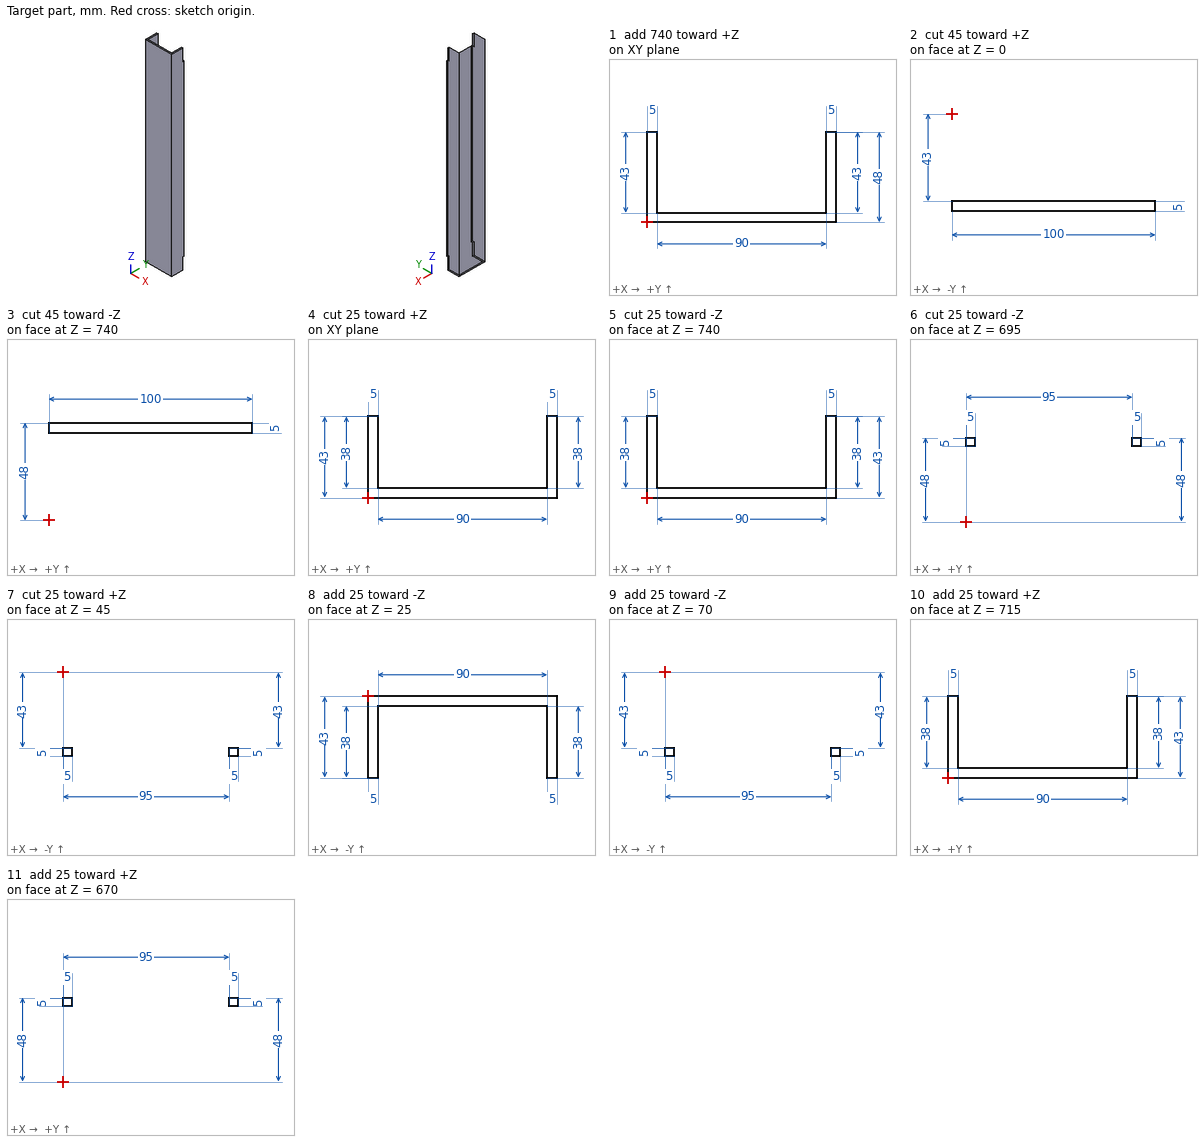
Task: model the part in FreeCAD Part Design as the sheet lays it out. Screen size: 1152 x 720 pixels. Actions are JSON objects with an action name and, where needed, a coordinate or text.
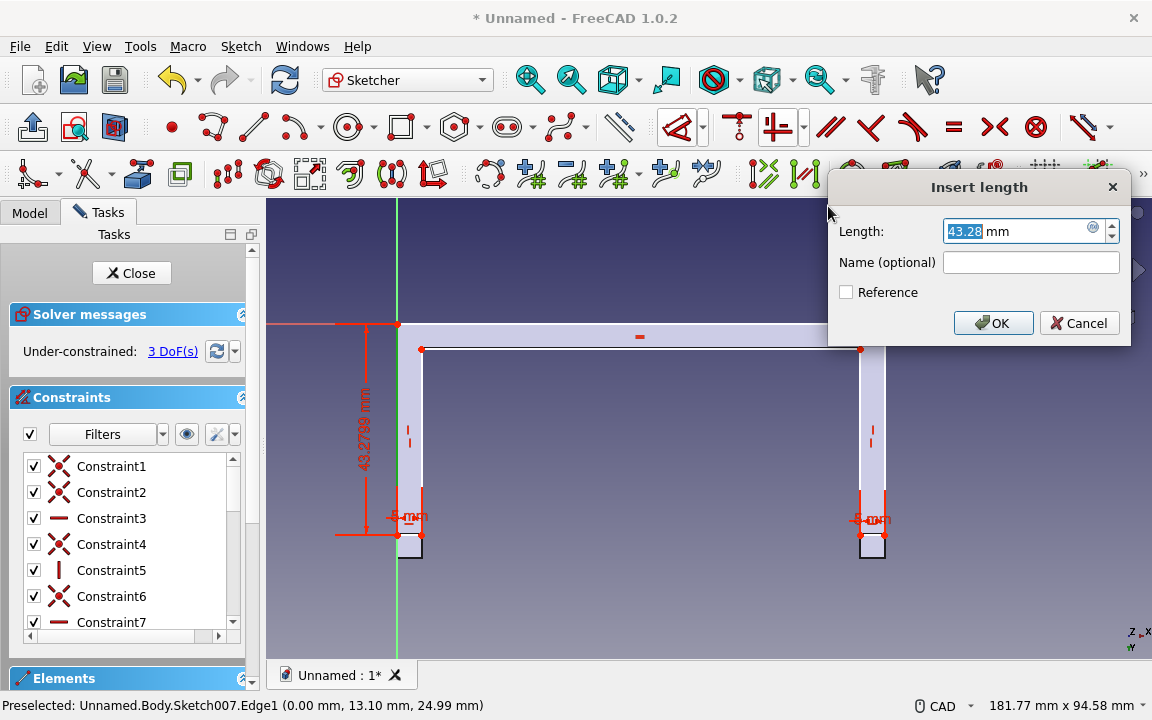
{"action": "type", "text": "43"}
{"action": "key", "text": "Return"}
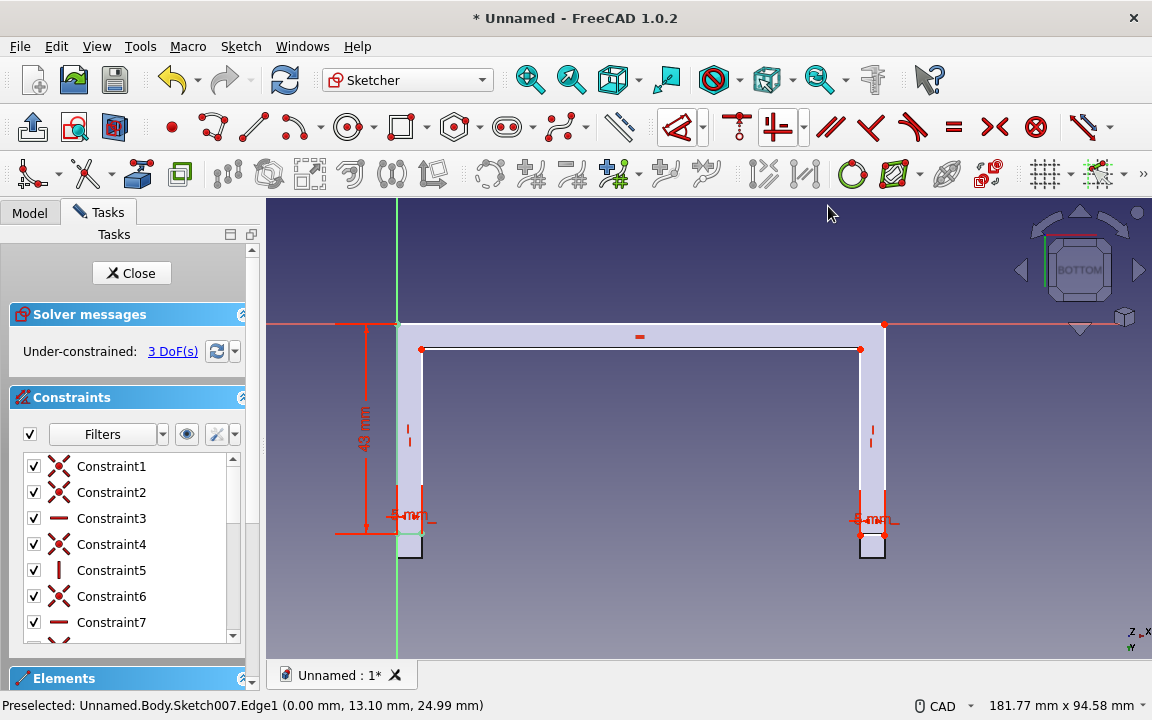
{"action": "left_click", "coordinate": [422, 478]}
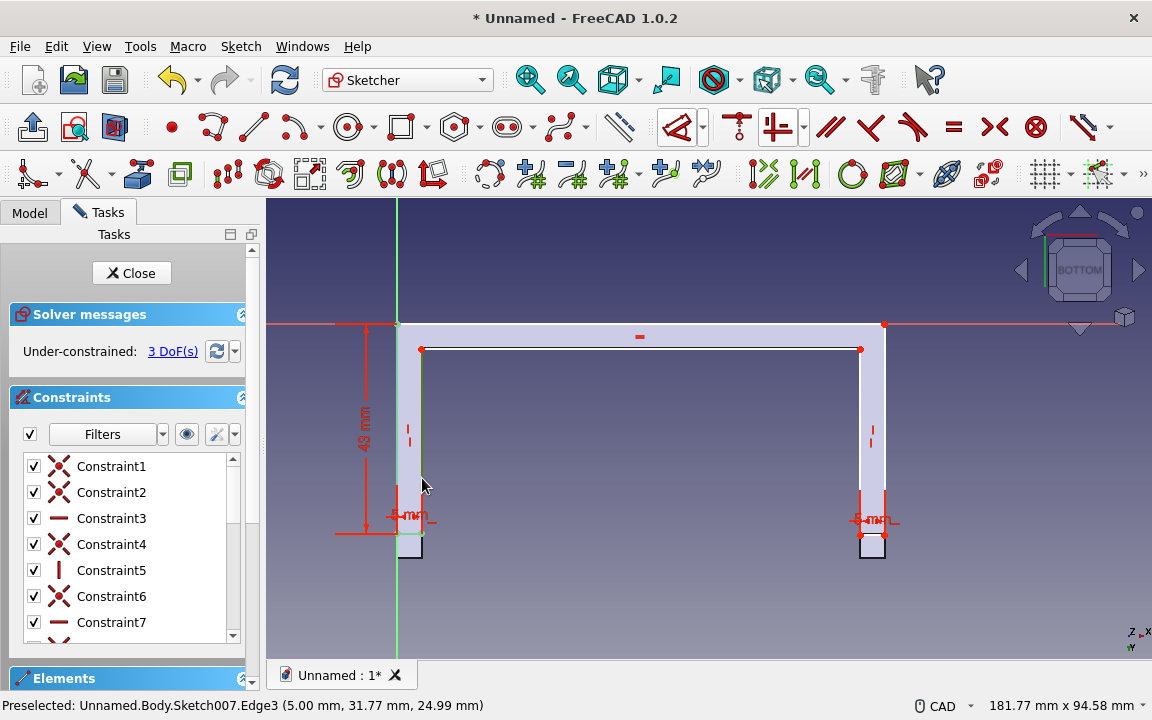
{"action": "left_click", "coordinate": [702, 128]}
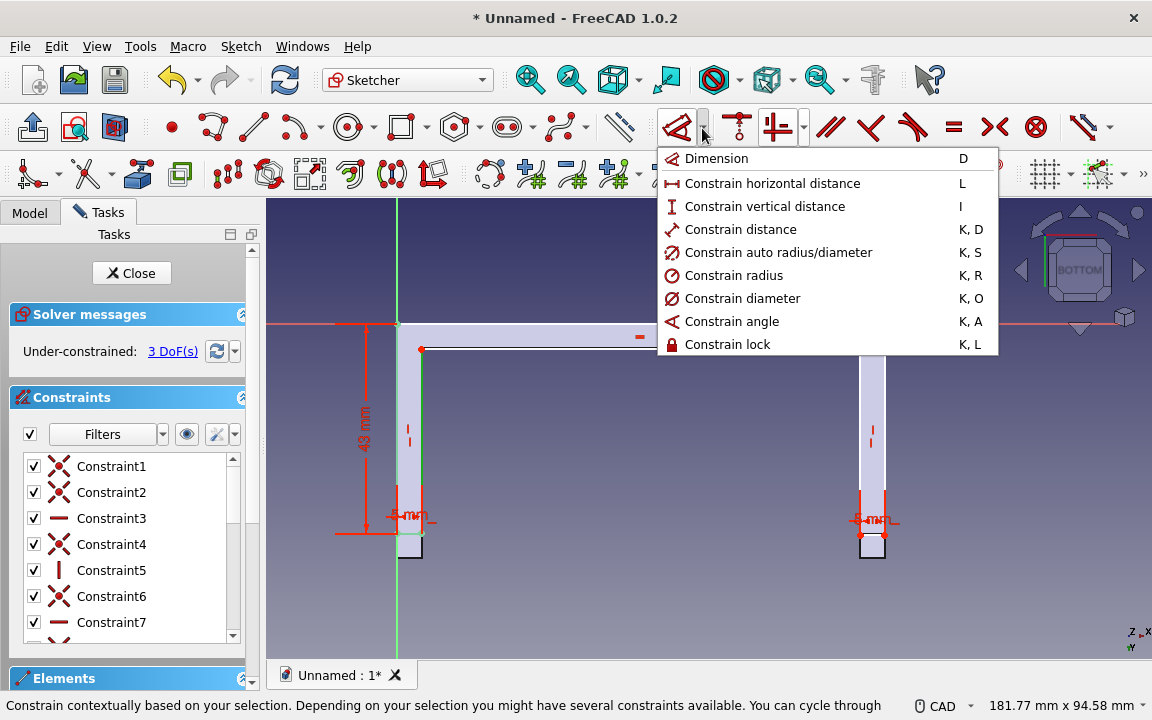
{"action": "left_click", "coordinate": [828, 206]}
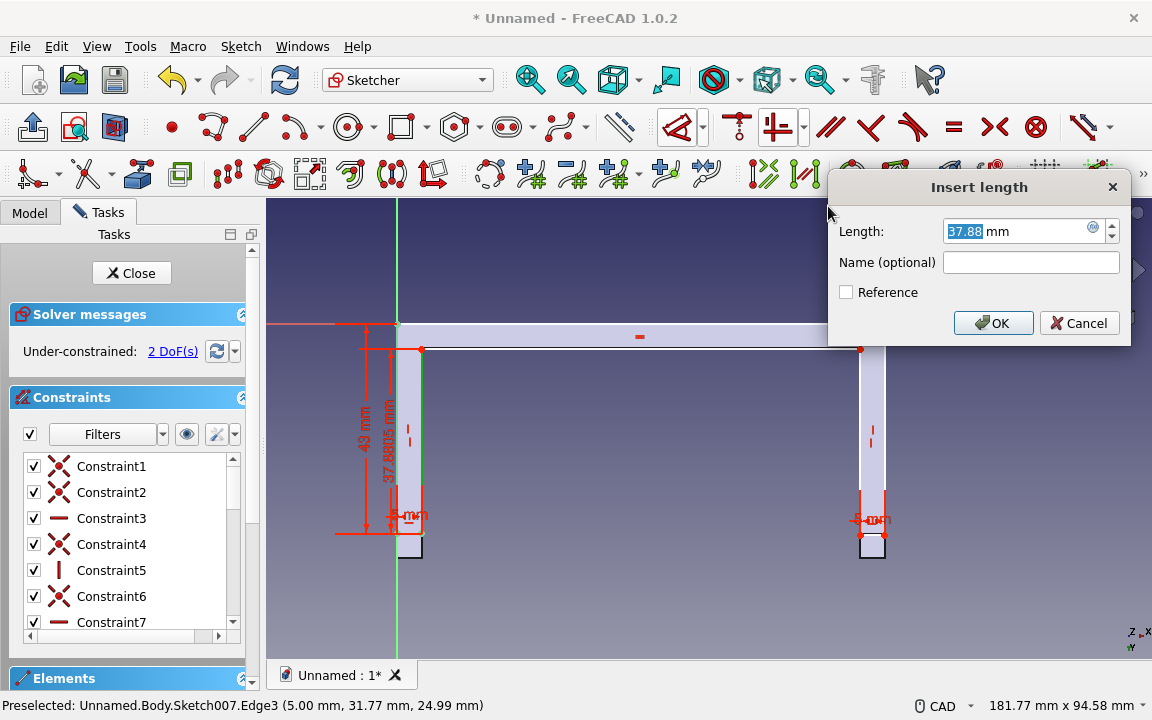
{"action": "type", "text": "38"}
{"action": "key", "text": "Return"}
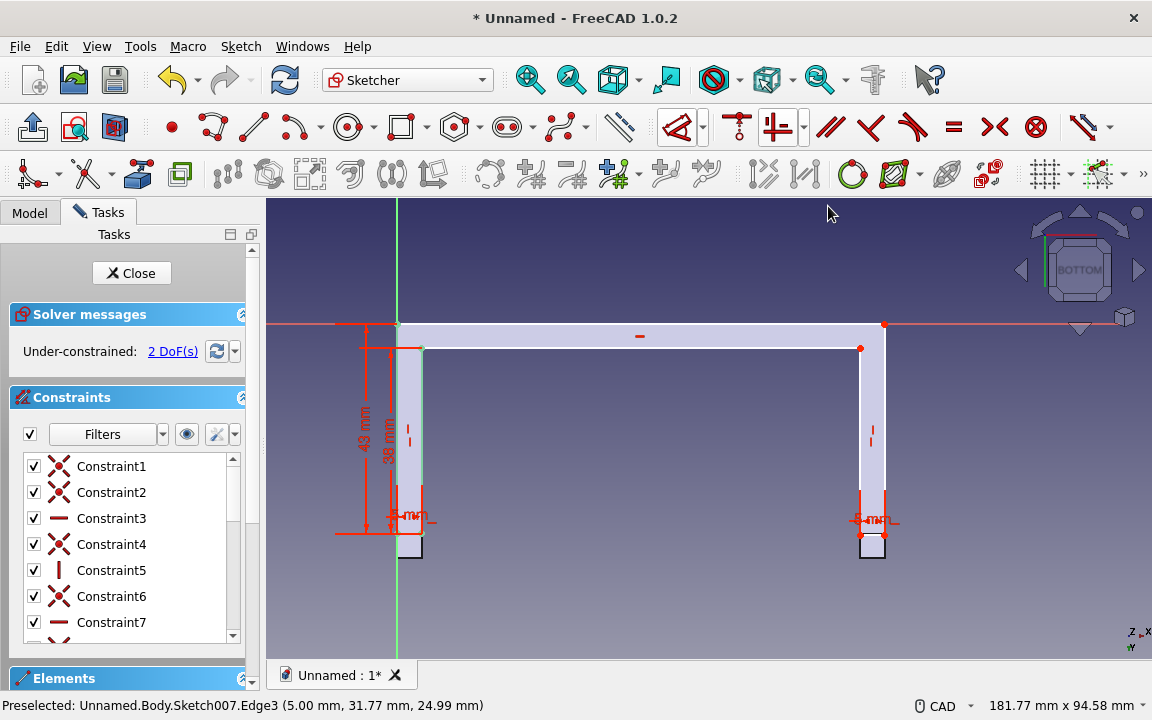
{"action": "left_click", "coordinate": [553, 348]}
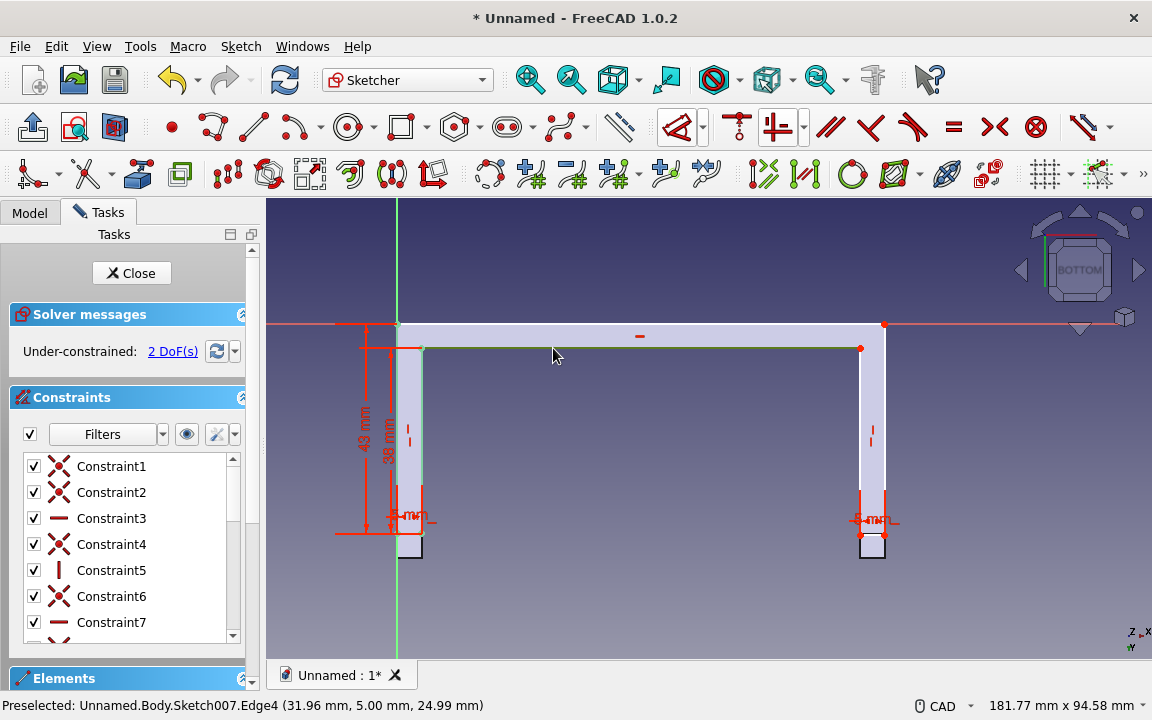
{"action": "left_click", "coordinate": [702, 128]}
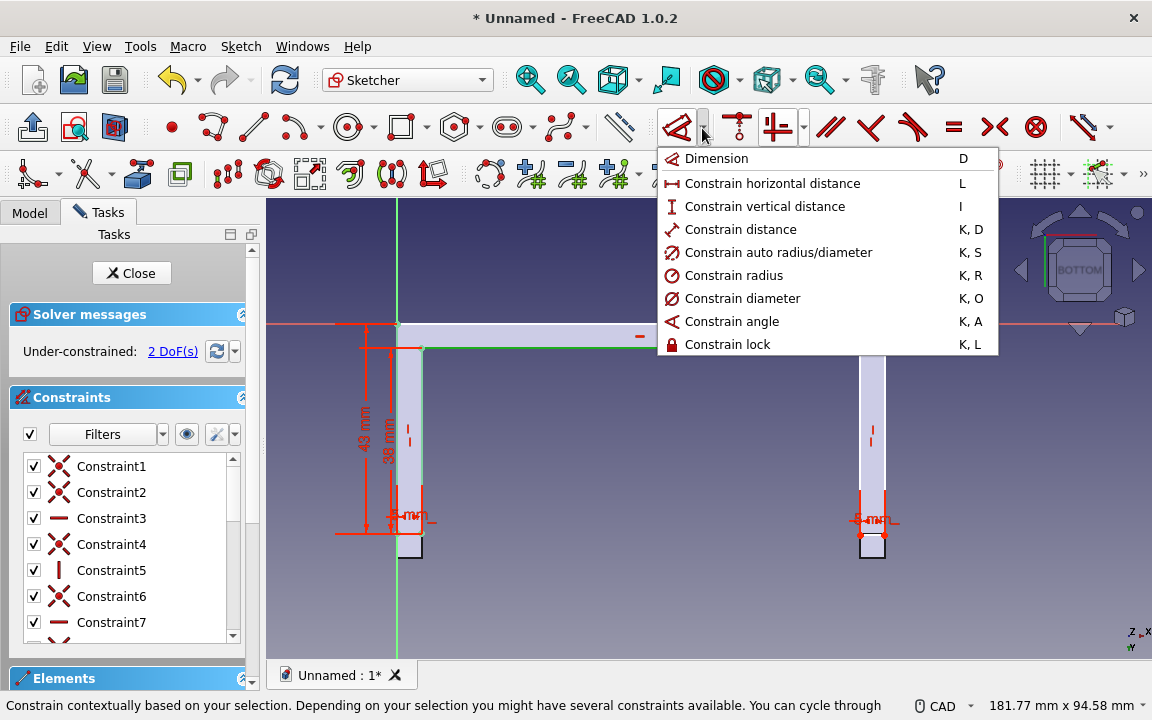
{"action": "left_click", "coordinate": [828, 184]}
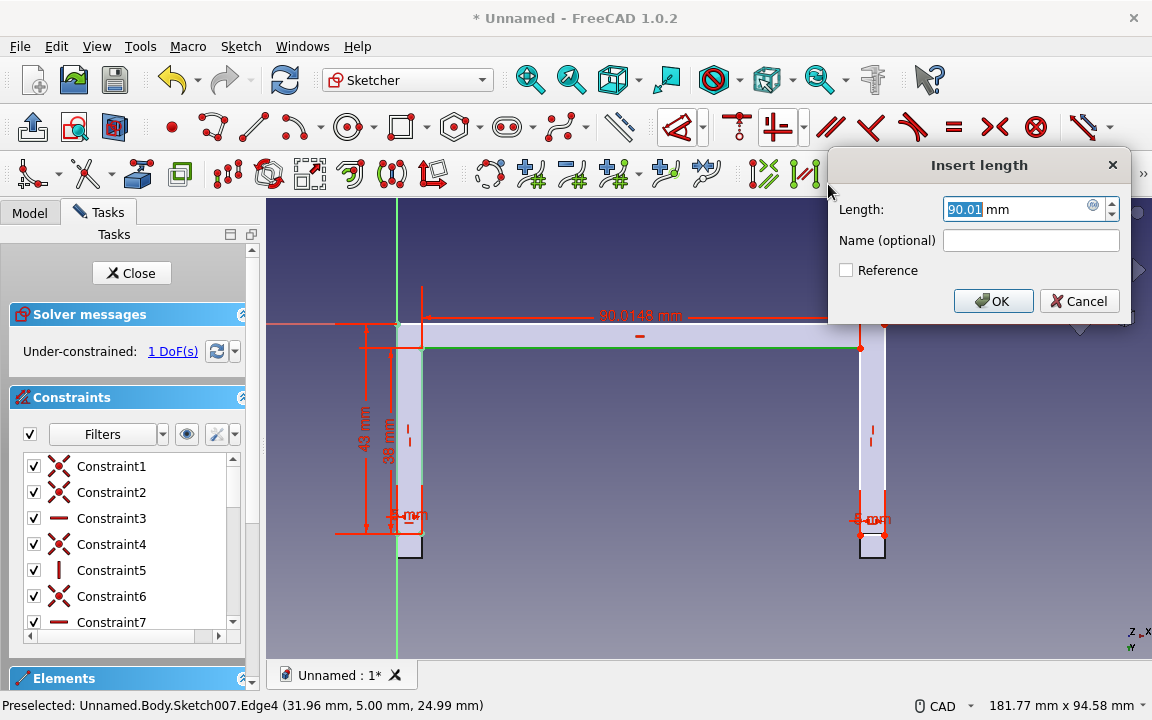
{"action": "type", "text": "90"}
{"action": "key", "text": "Return"}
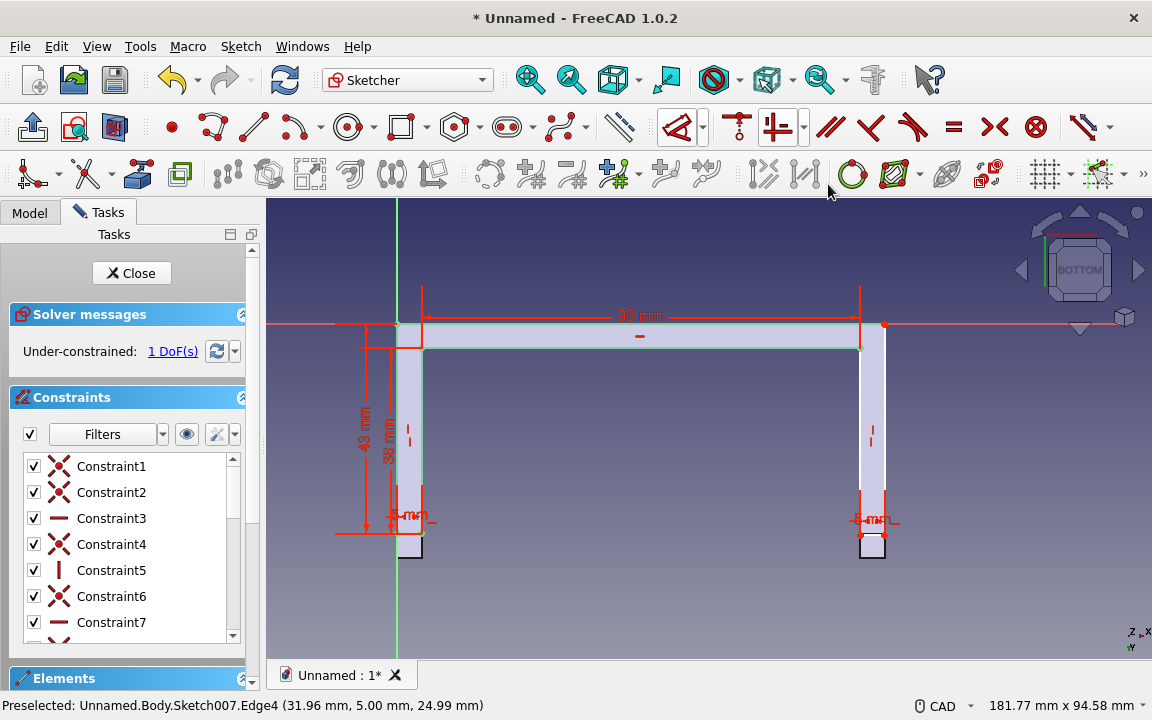
{"action": "left_click", "coordinate": [860, 404]}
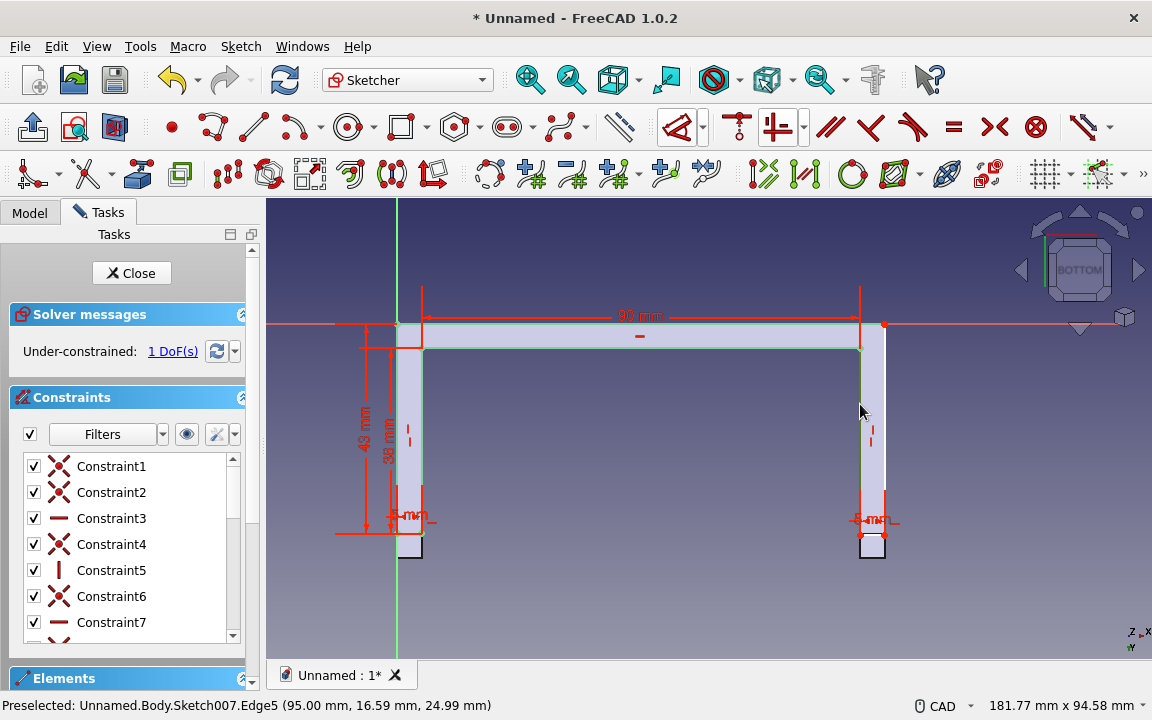
{"action": "left_click", "coordinate": [702, 128]}